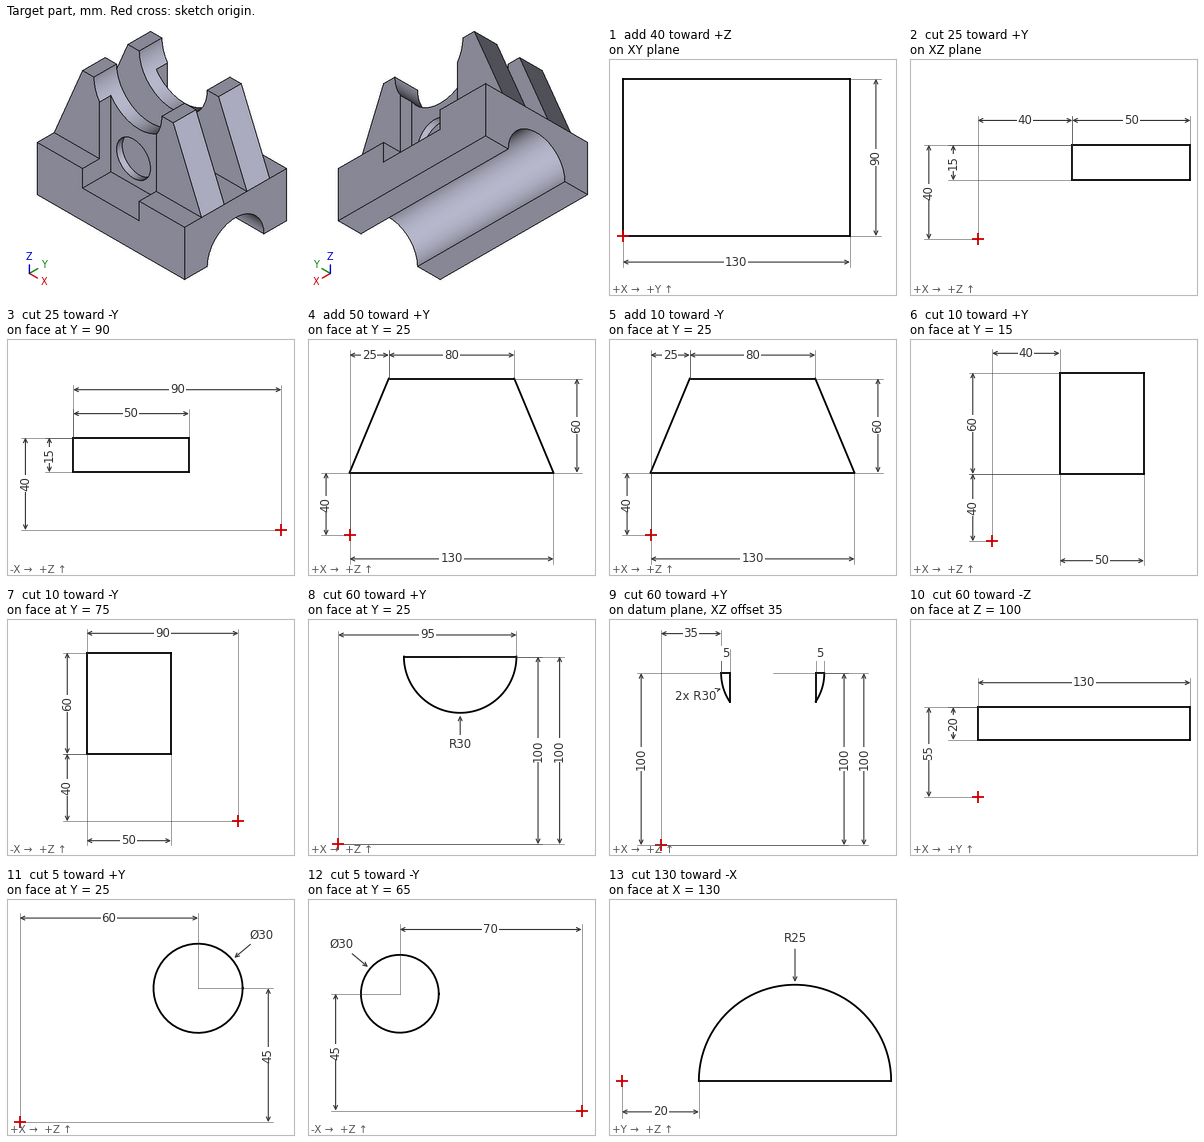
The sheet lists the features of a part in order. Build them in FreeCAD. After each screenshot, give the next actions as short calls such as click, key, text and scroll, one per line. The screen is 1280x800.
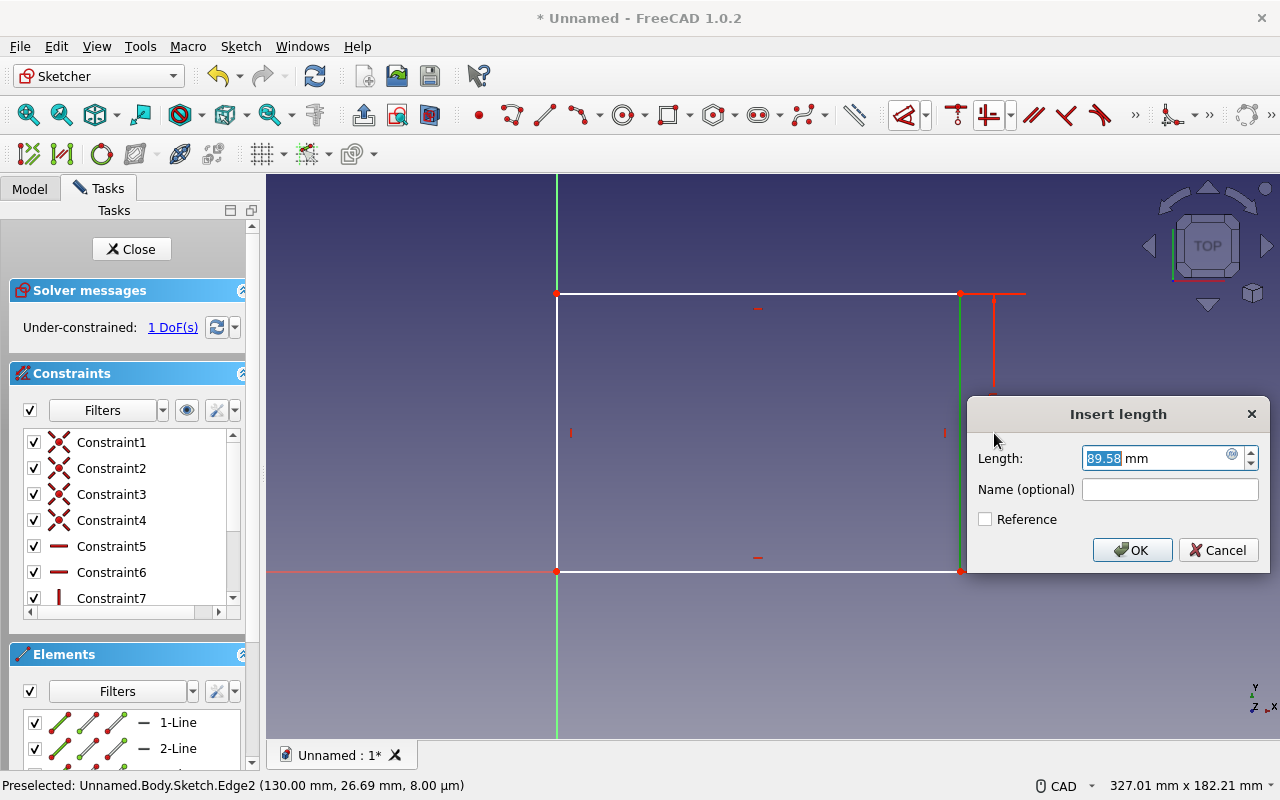
text(90)
key(Return)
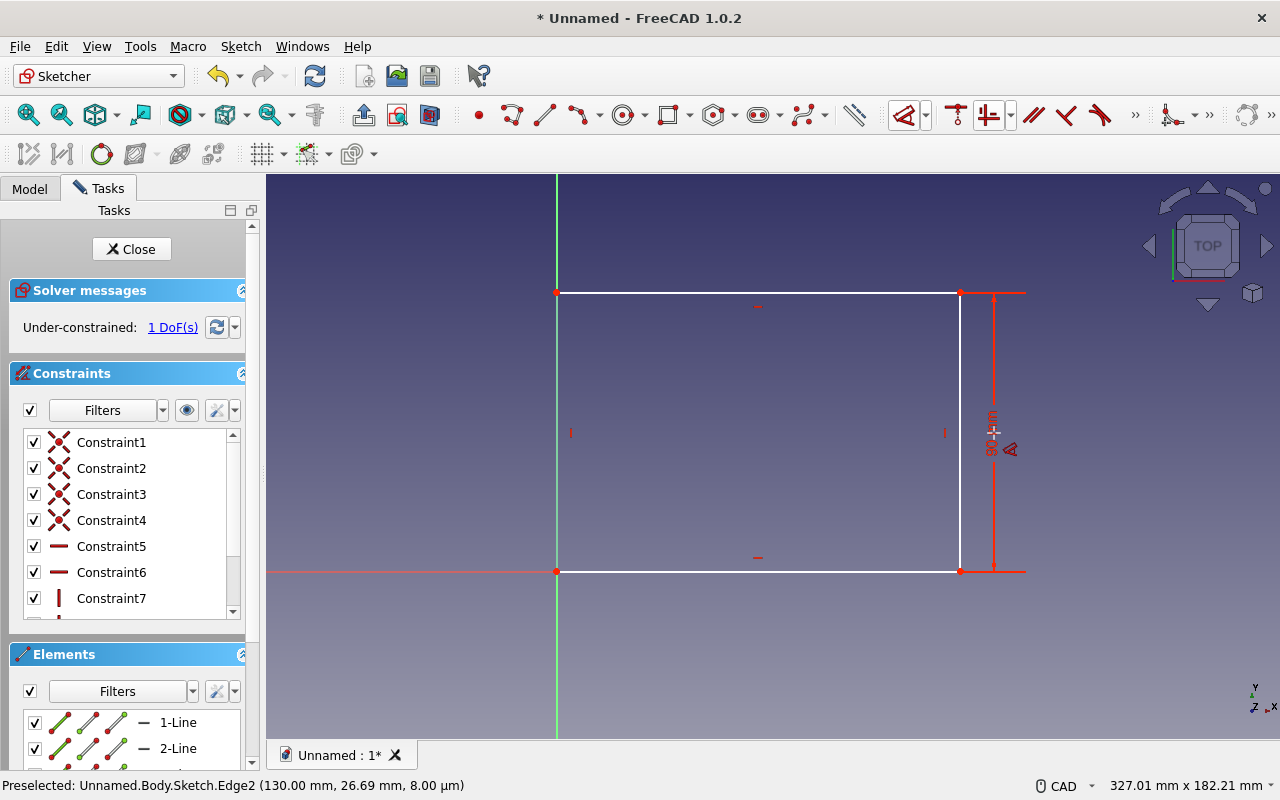
click(678, 572)
click(758, 606)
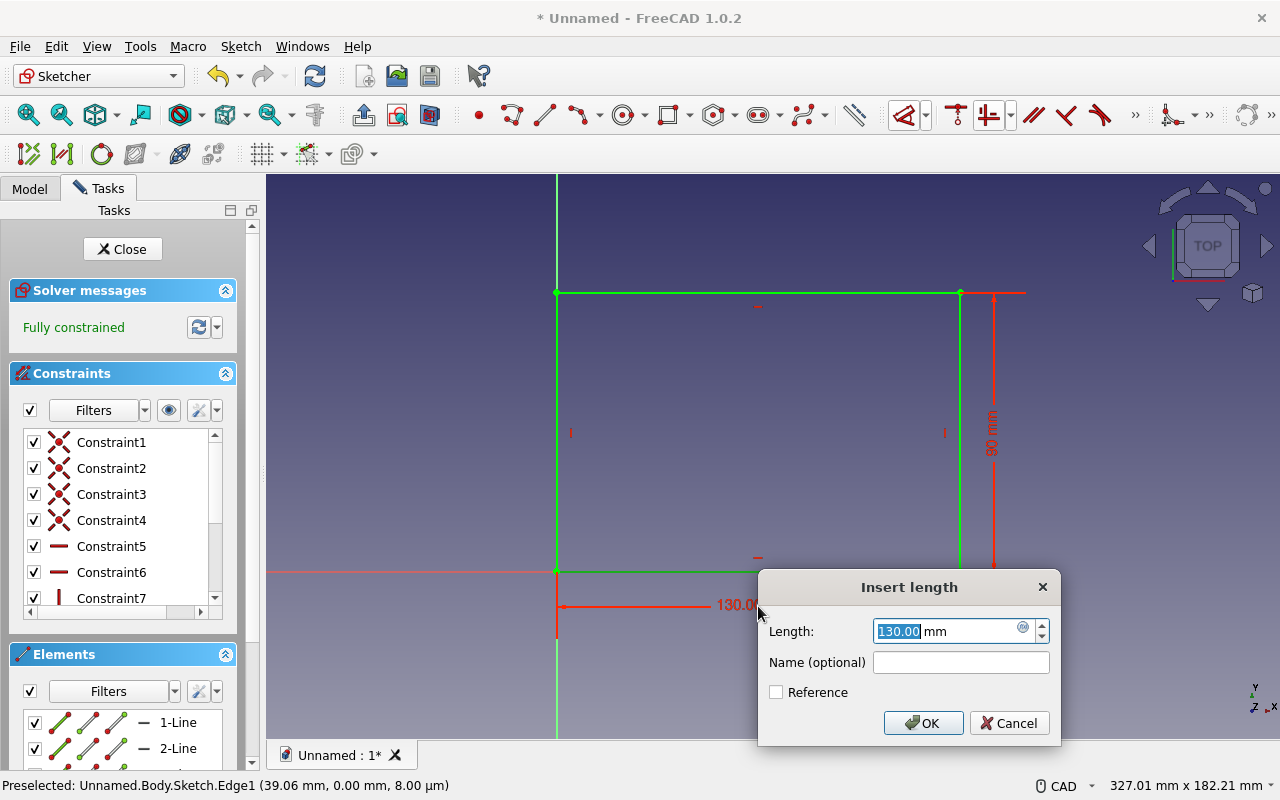
text(130)
key(Return)
key(Escape)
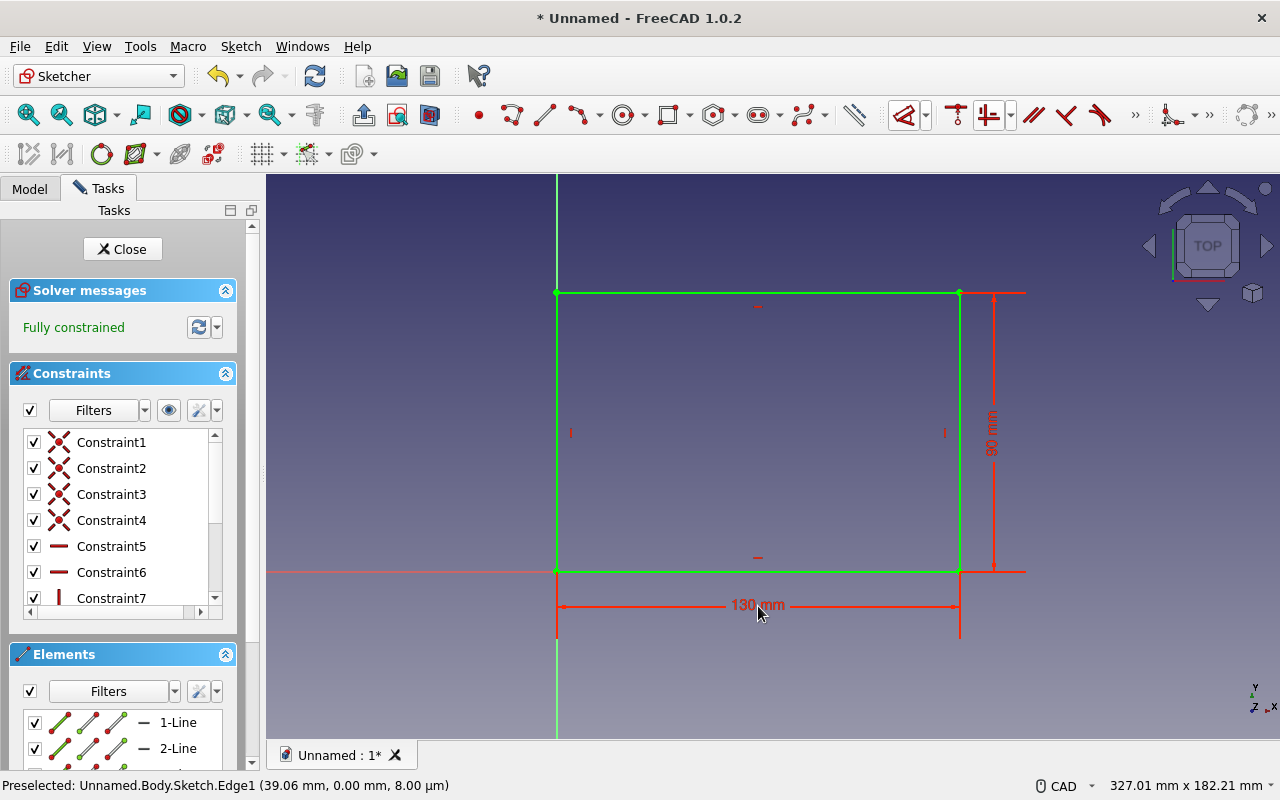
click(123, 249)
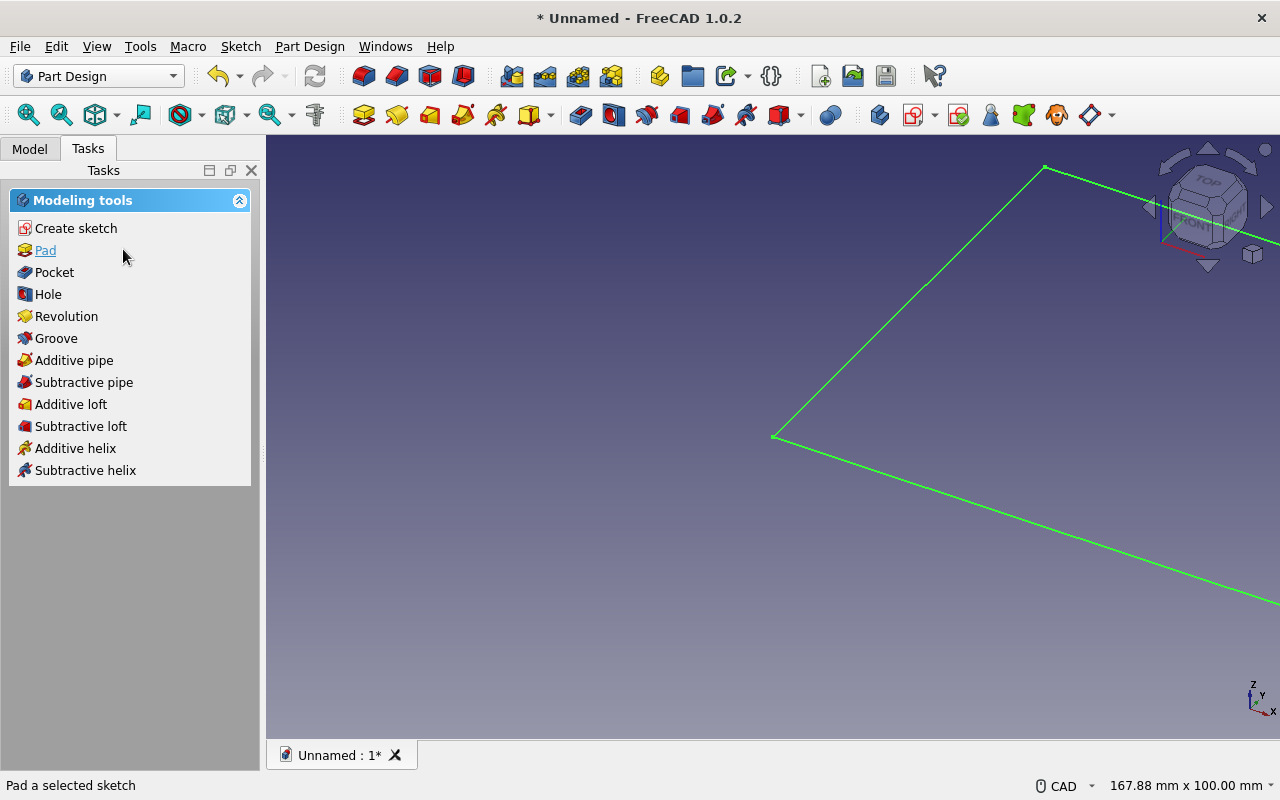
click(364, 116)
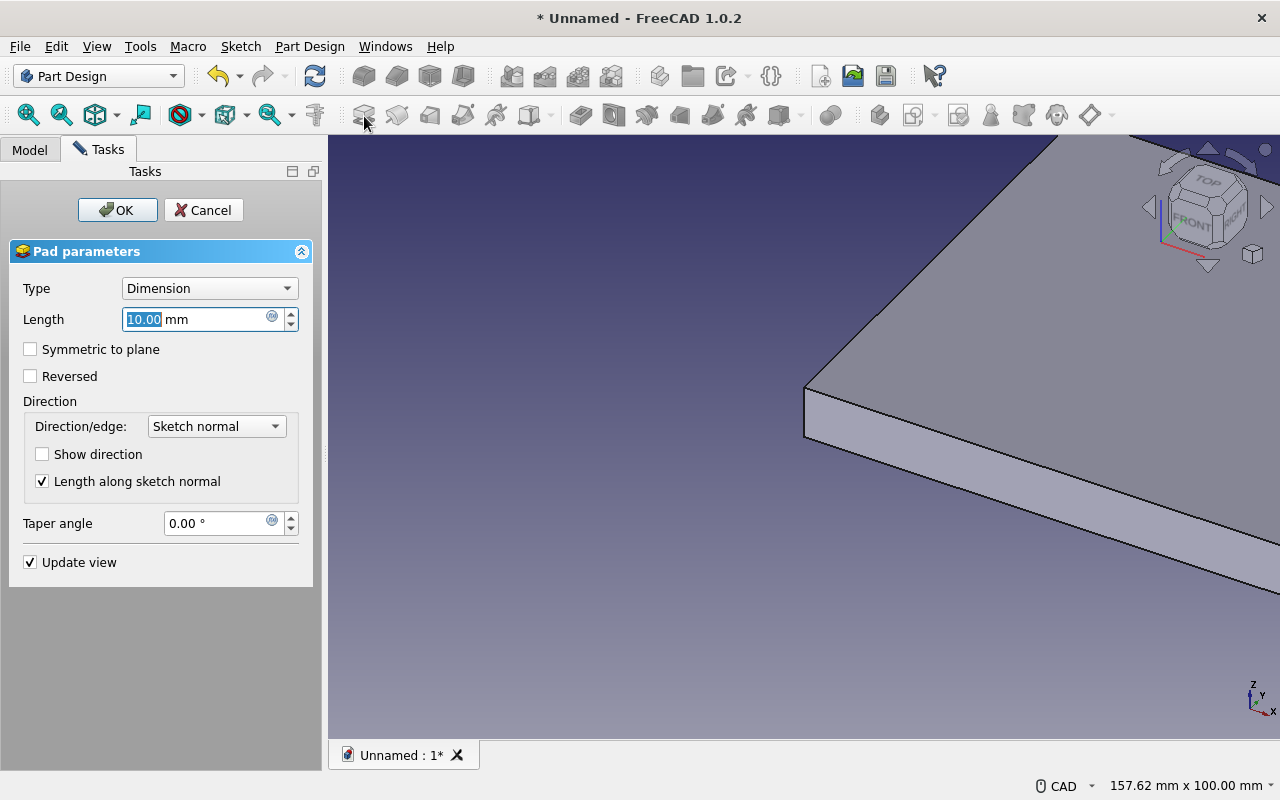
text(40)
key(Tab)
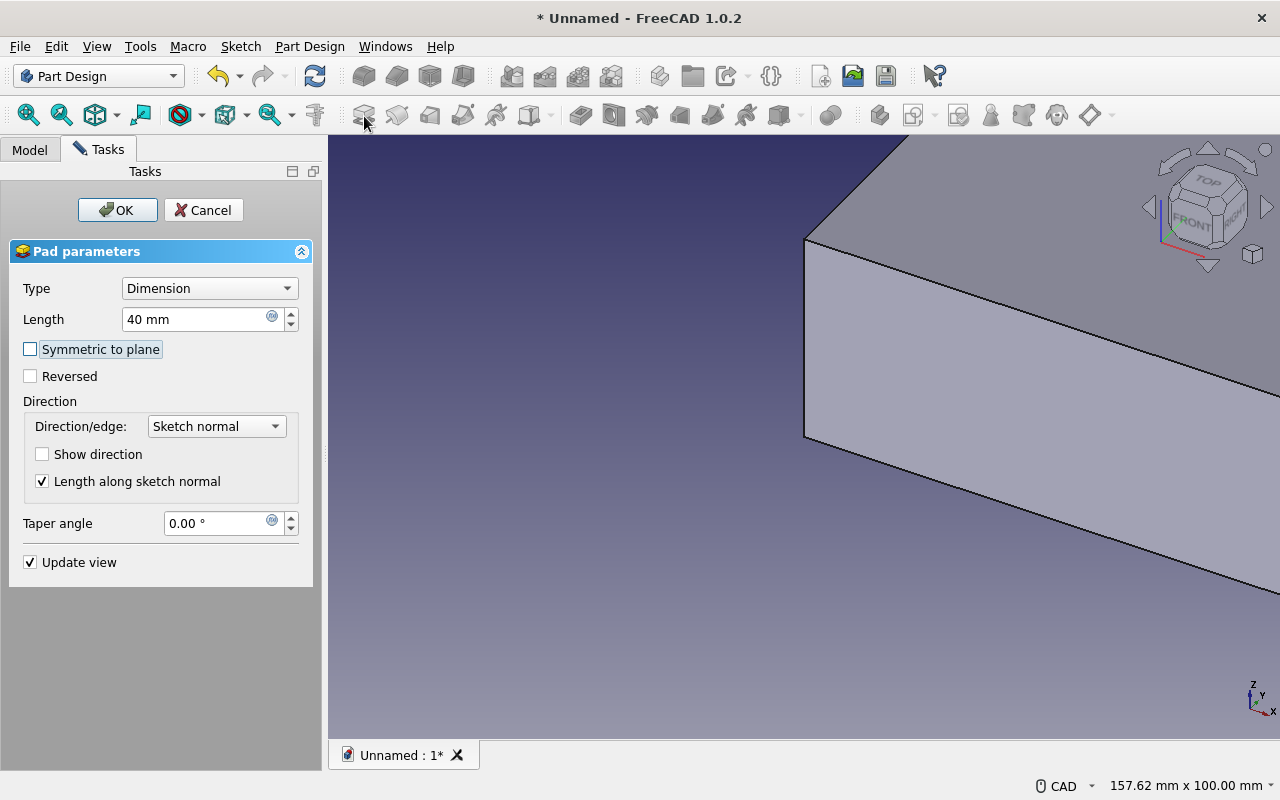
click(118, 210)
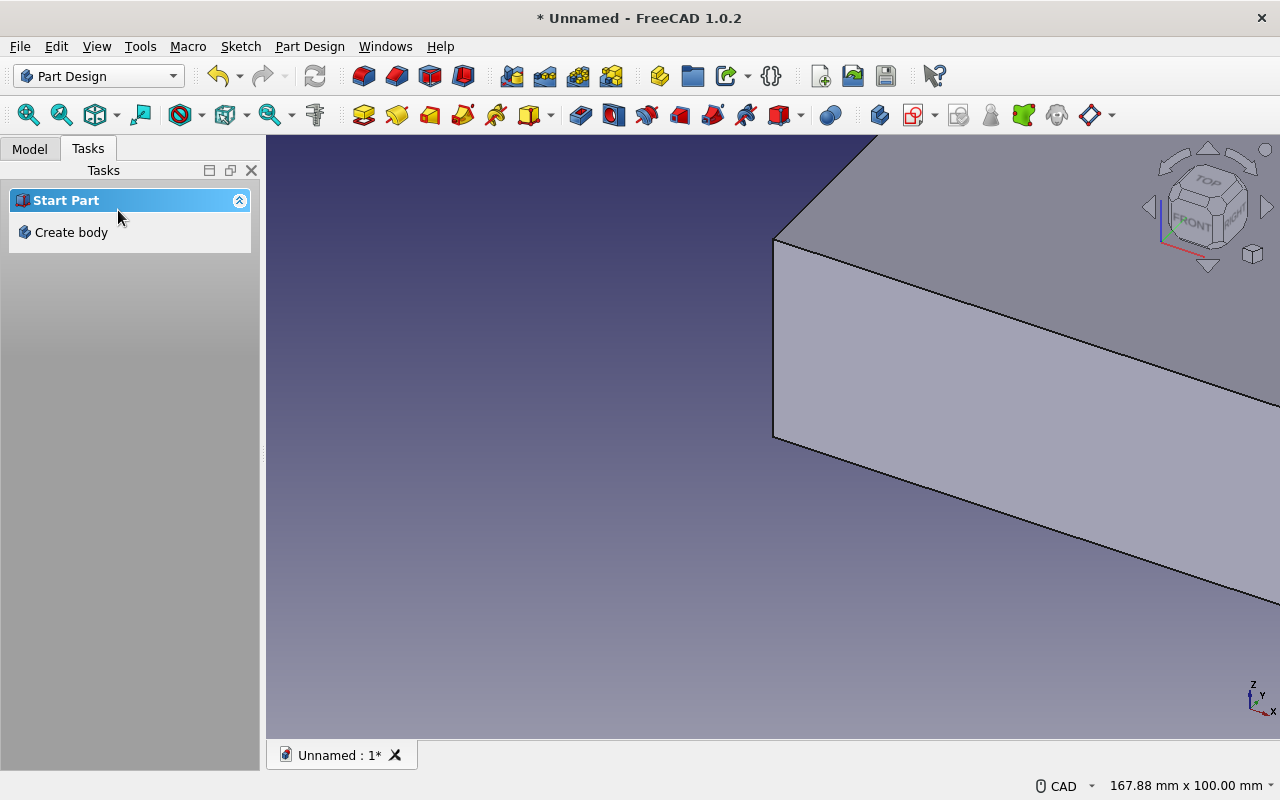
key(v)
key(f)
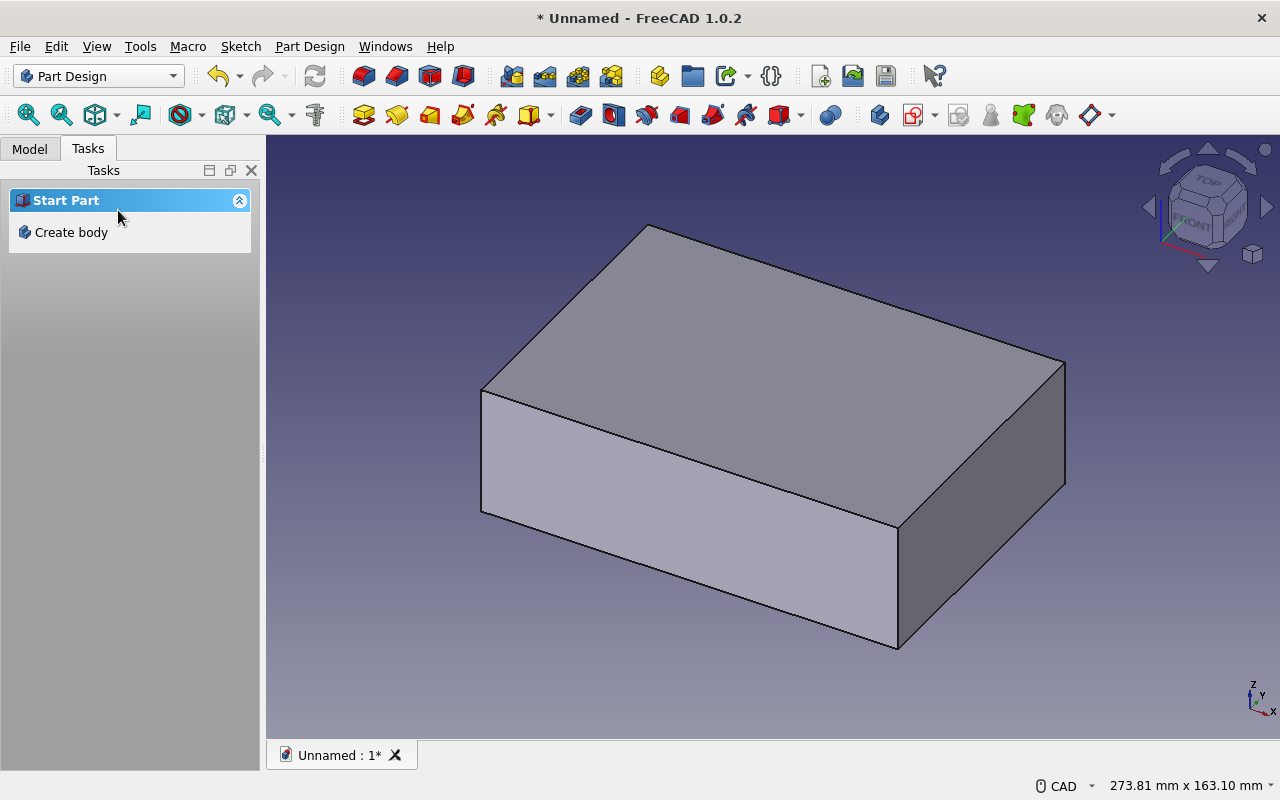
click(912, 116)